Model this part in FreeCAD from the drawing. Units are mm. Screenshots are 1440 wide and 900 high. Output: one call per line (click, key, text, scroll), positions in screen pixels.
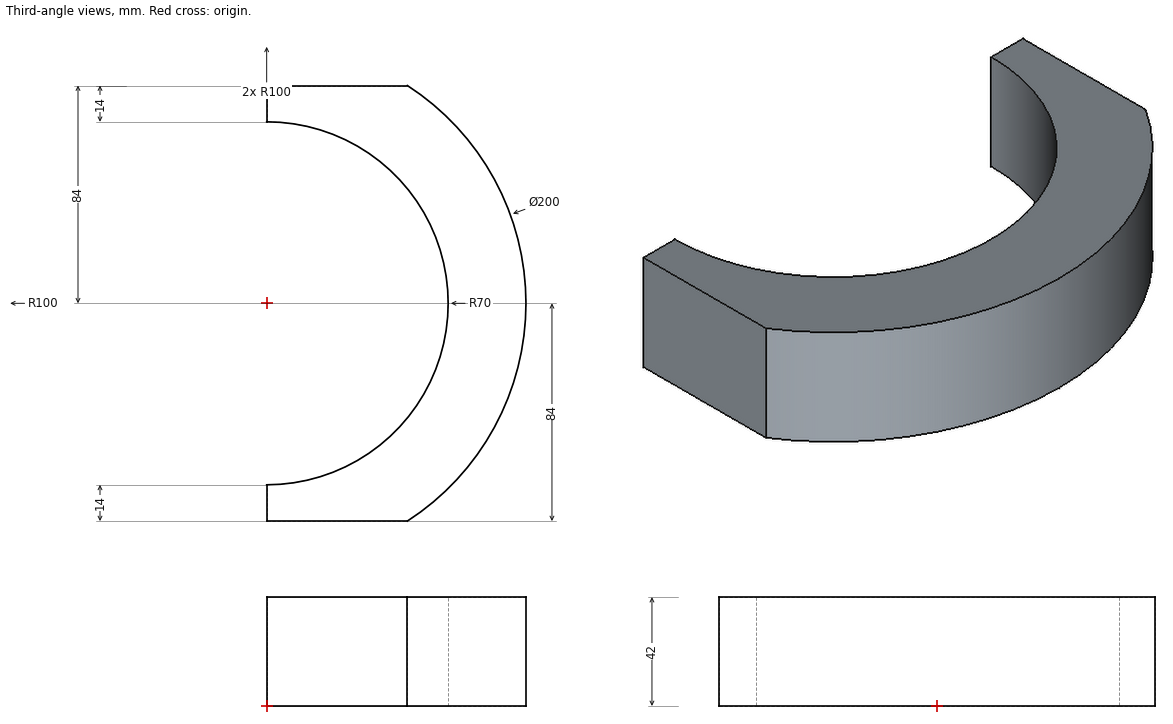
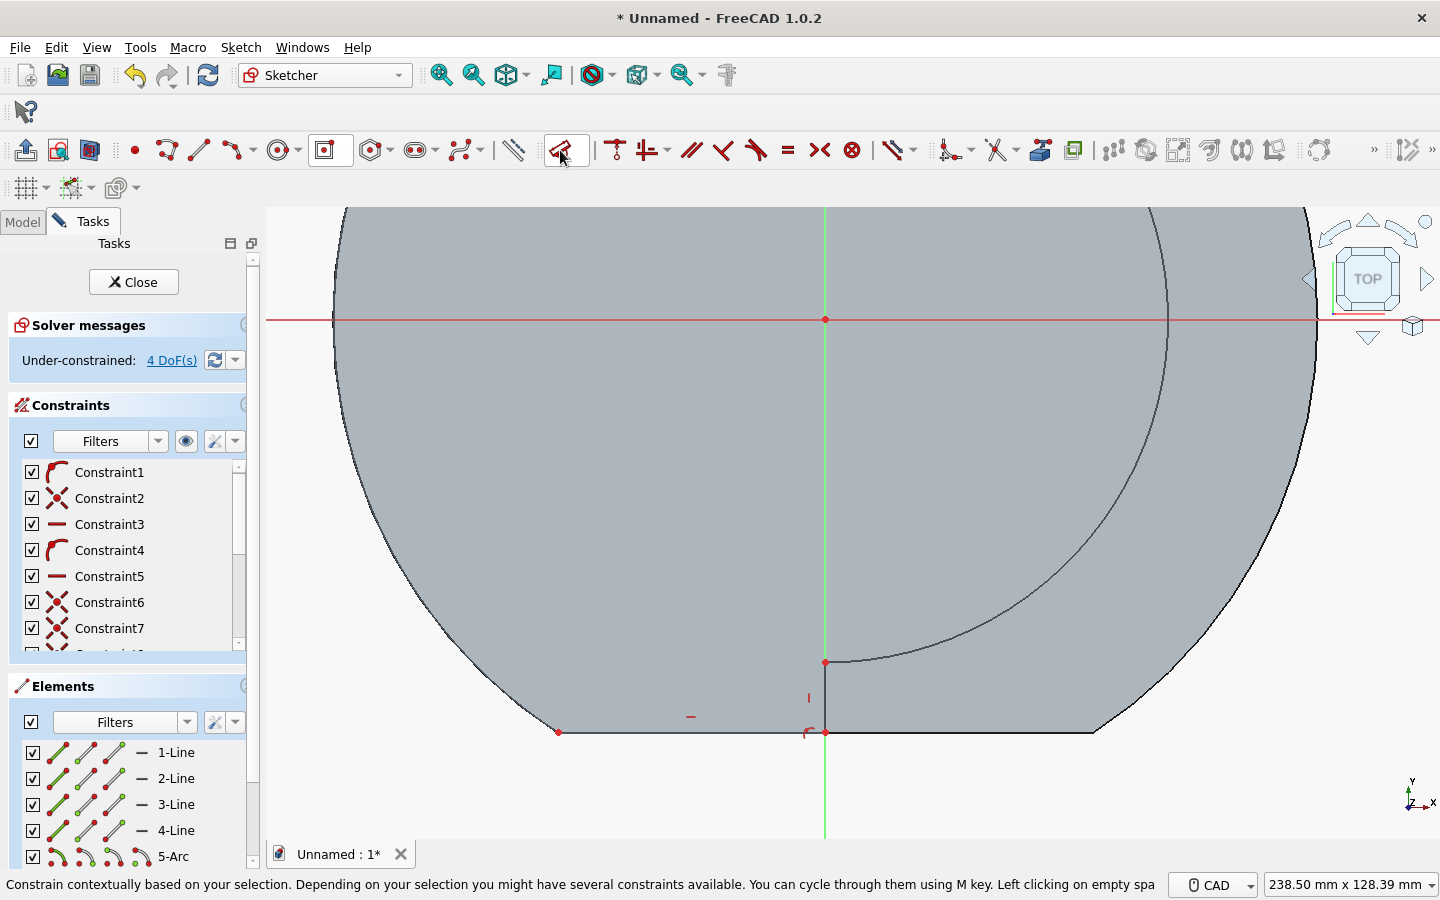
click(372, 511)
click(343, 523)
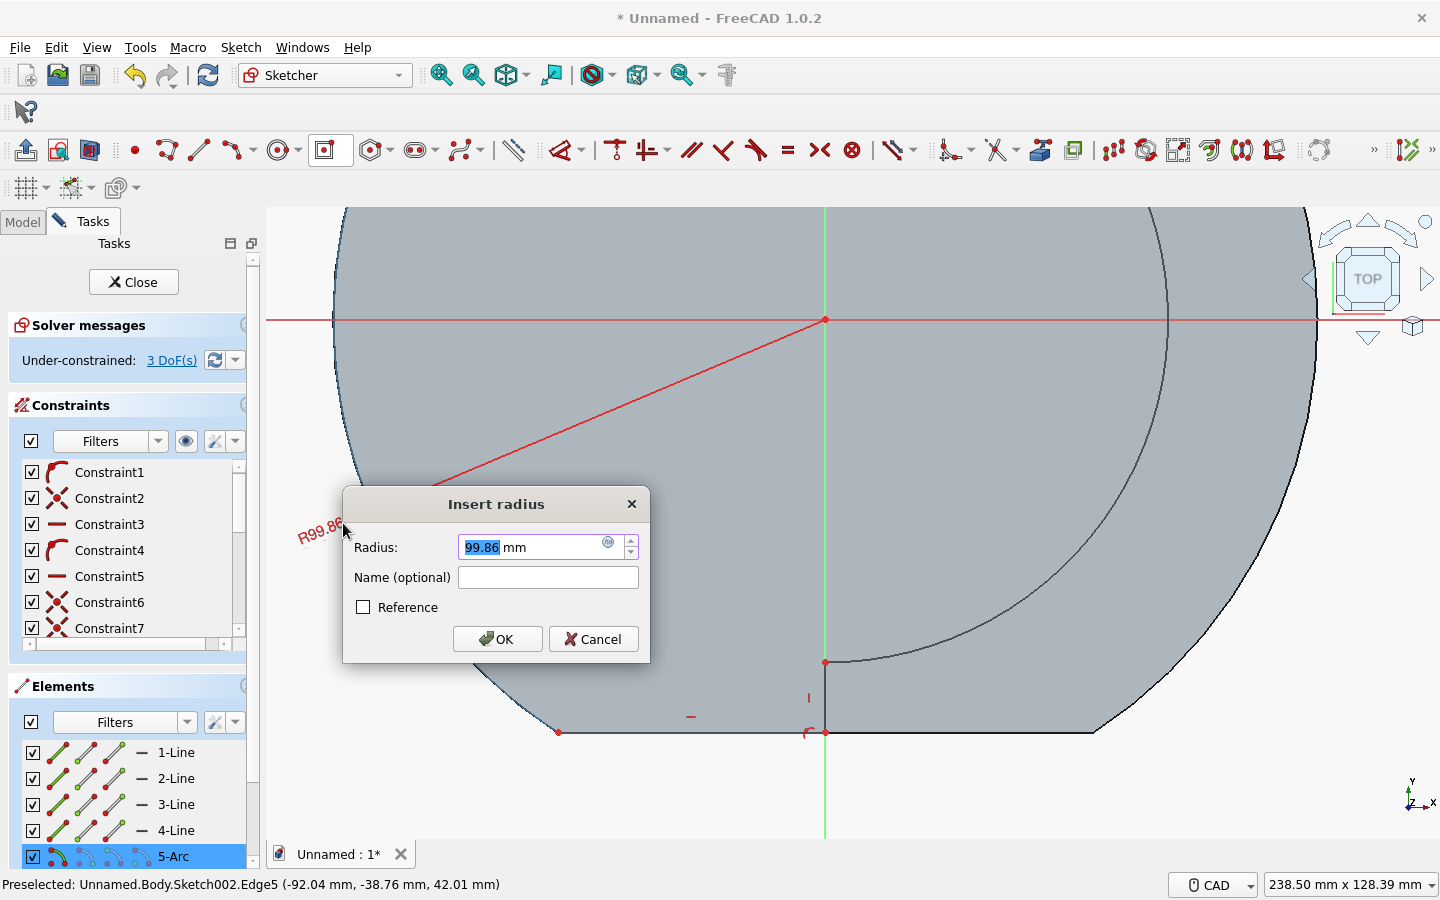
text(100)
key(Return)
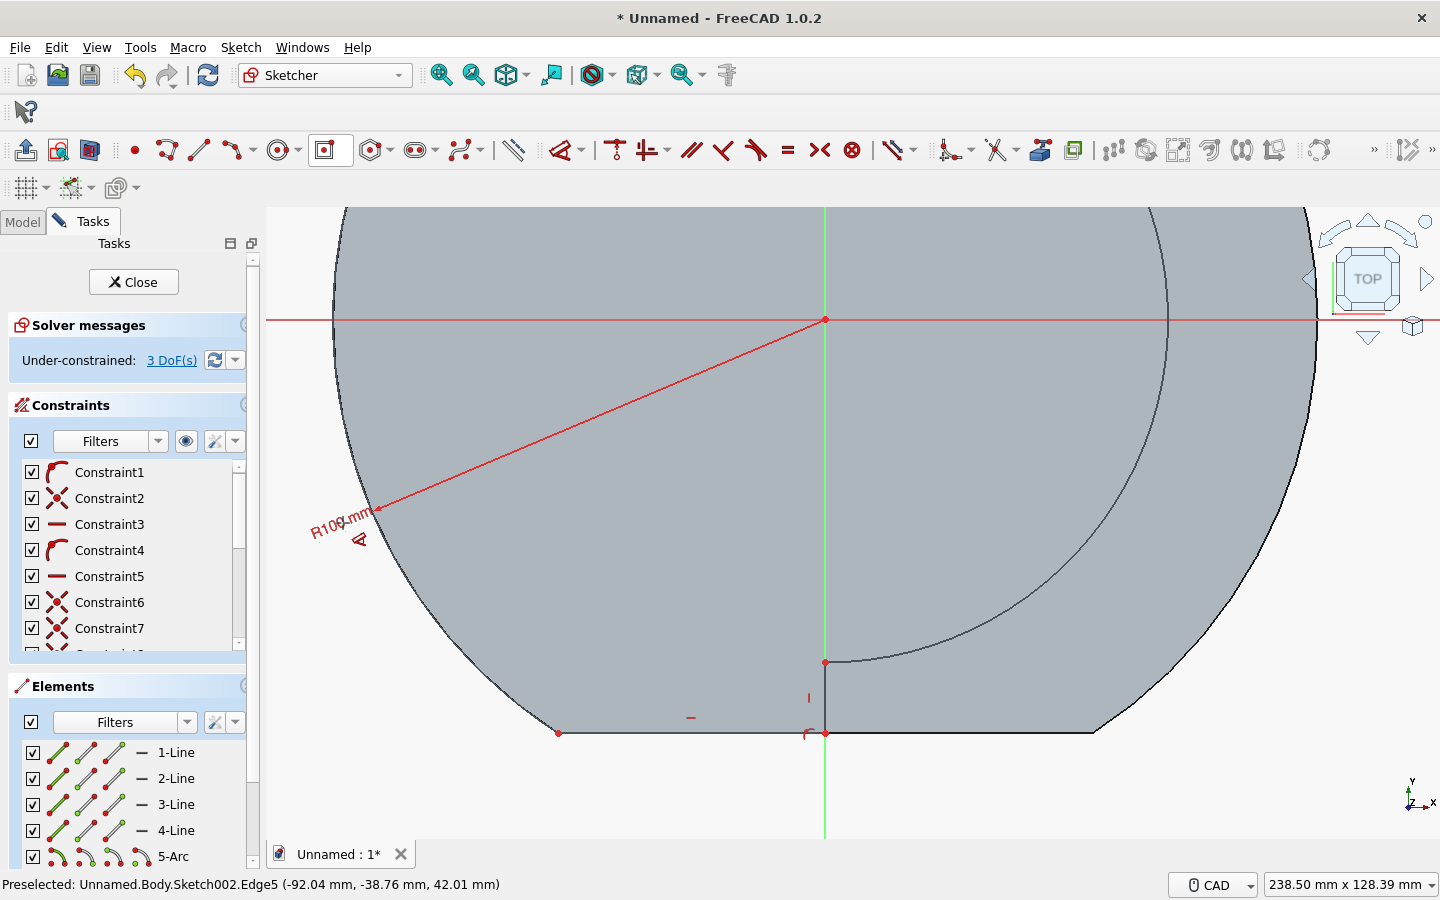
click(1103, 521)
click(1129, 540)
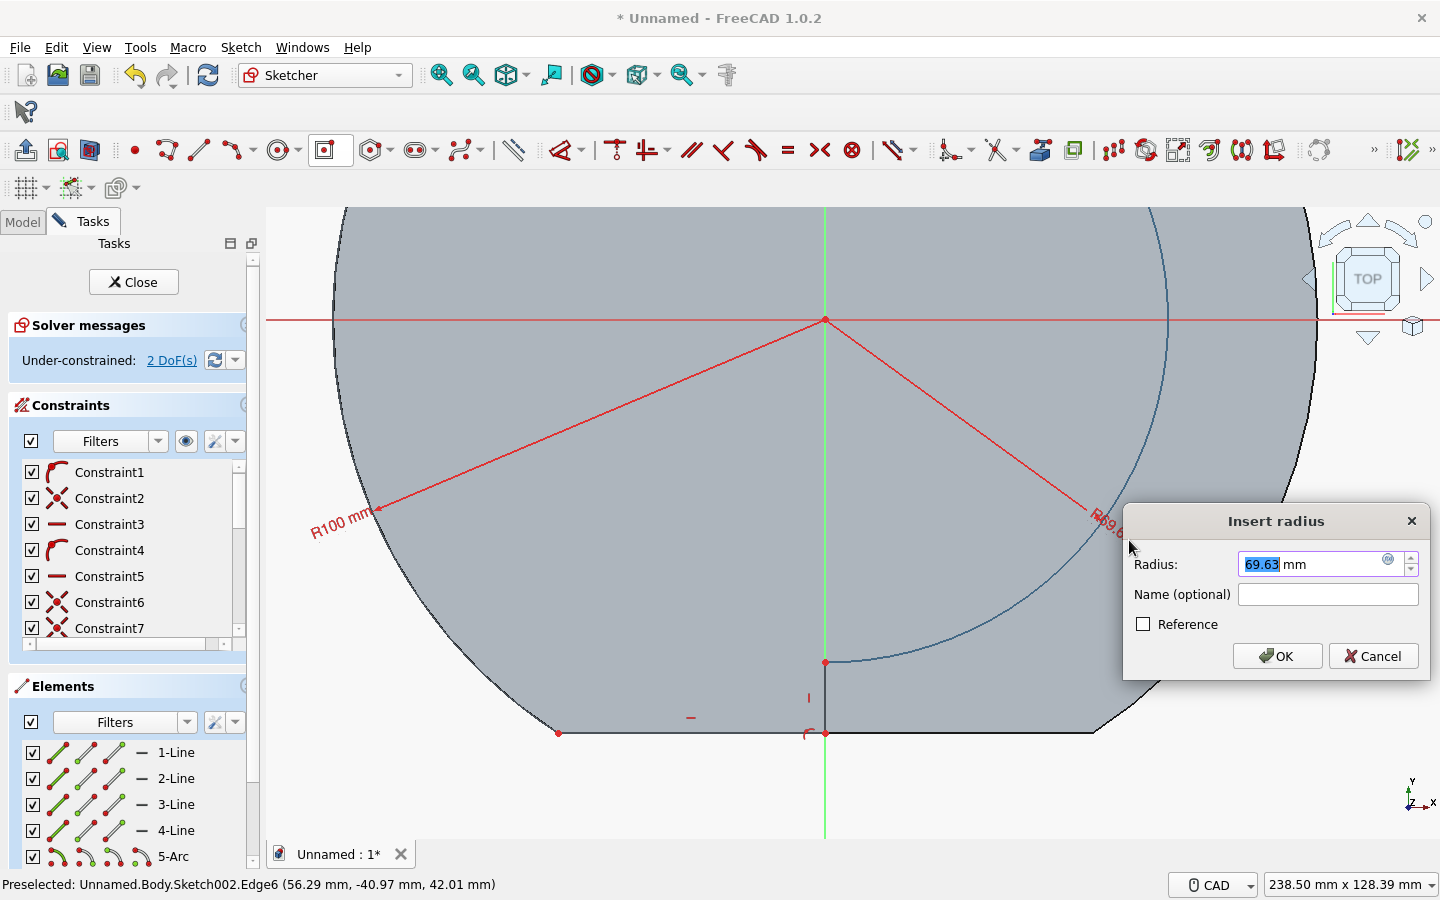
text(70)
key(Return)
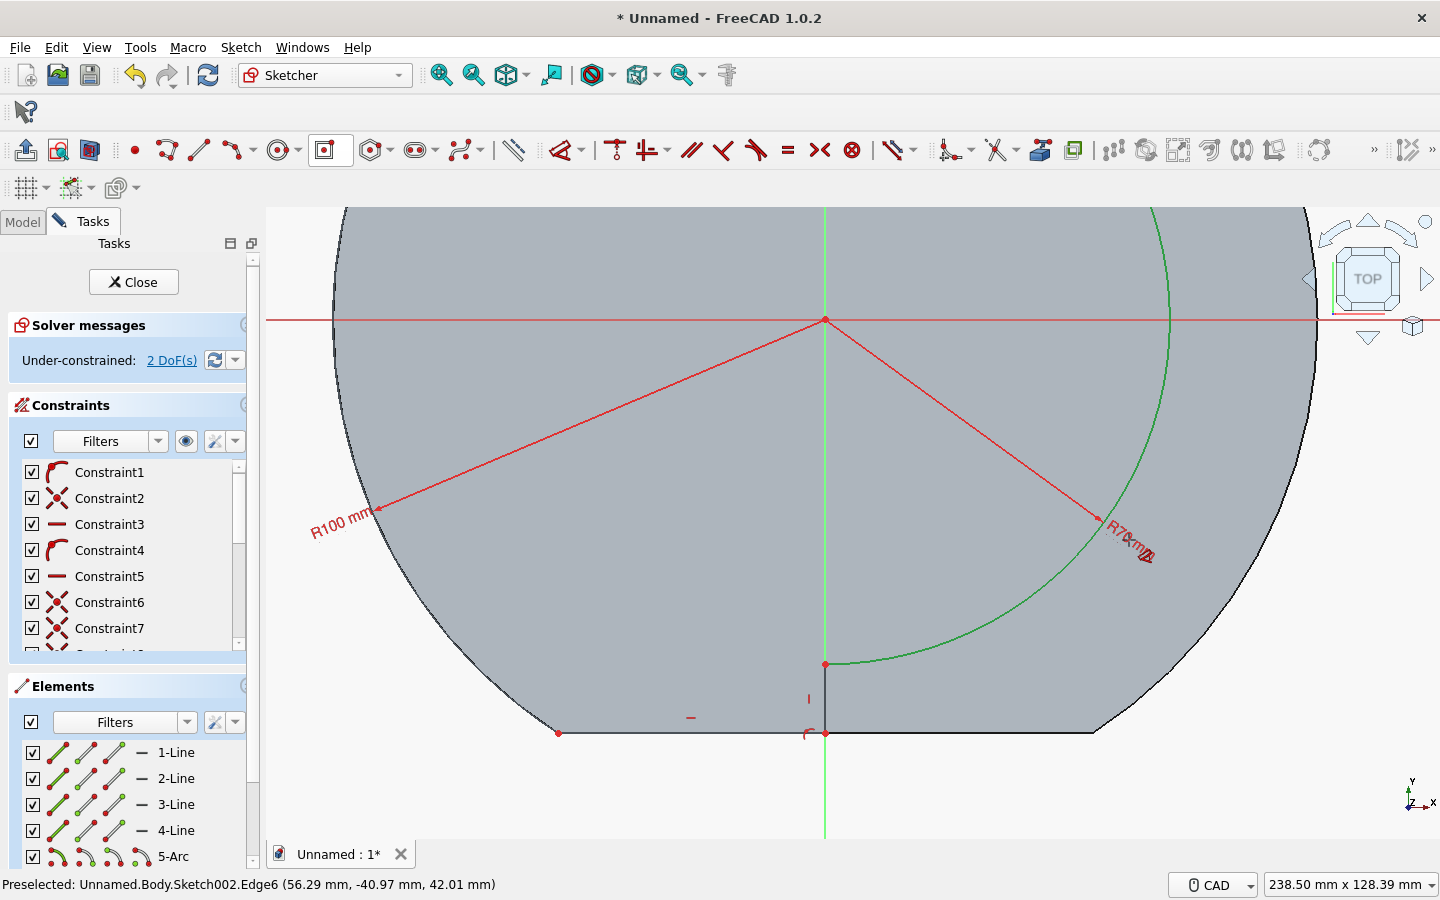
scroll(811, 689, down, 4)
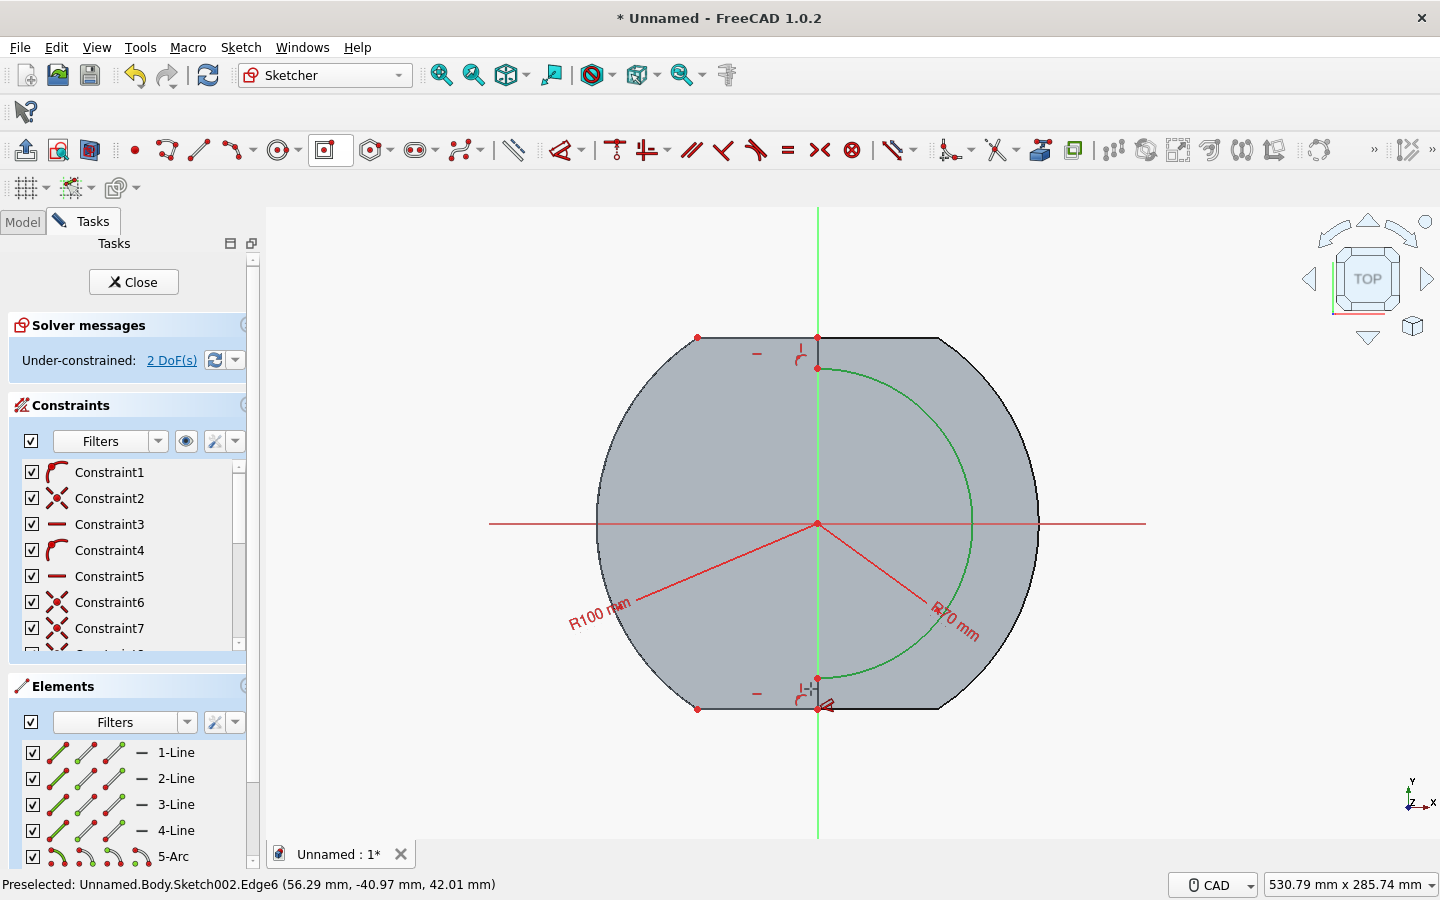
scroll(818, 359, up, 2)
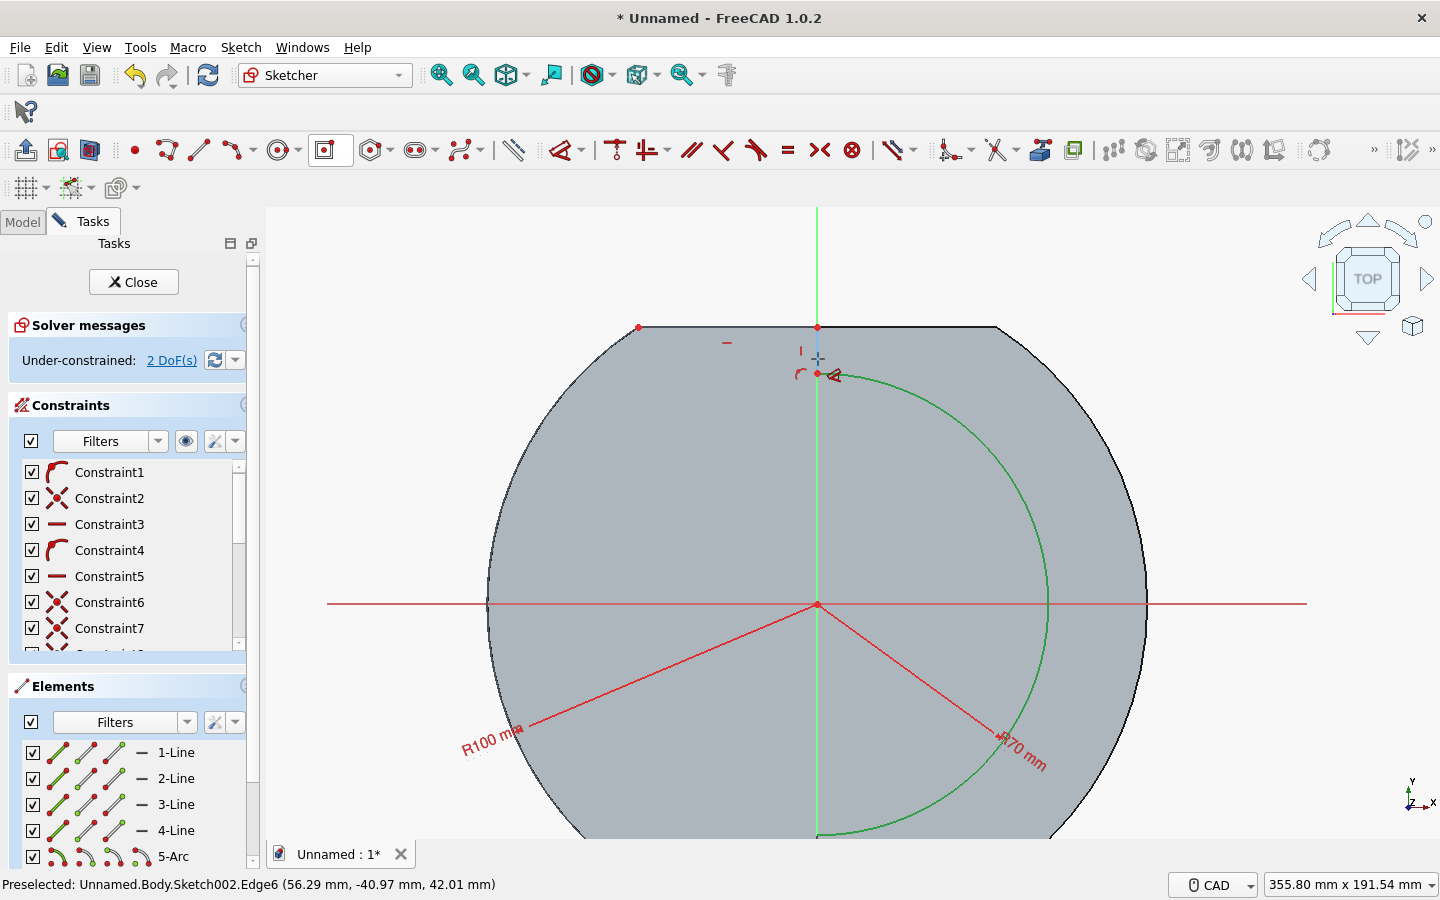
click(817, 360)
click(851, 350)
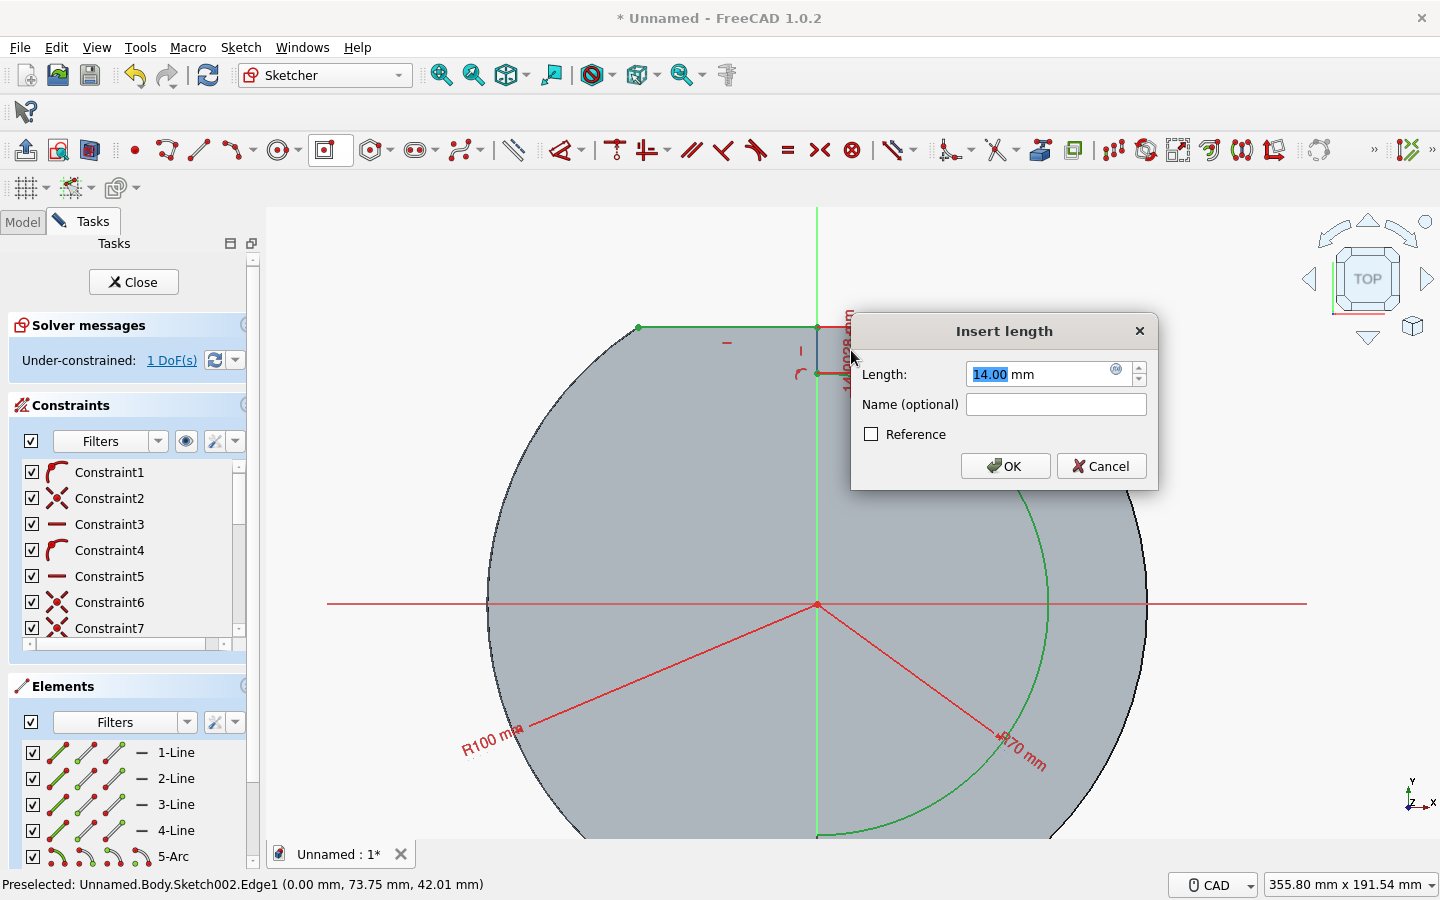
text(14)
key(Return)